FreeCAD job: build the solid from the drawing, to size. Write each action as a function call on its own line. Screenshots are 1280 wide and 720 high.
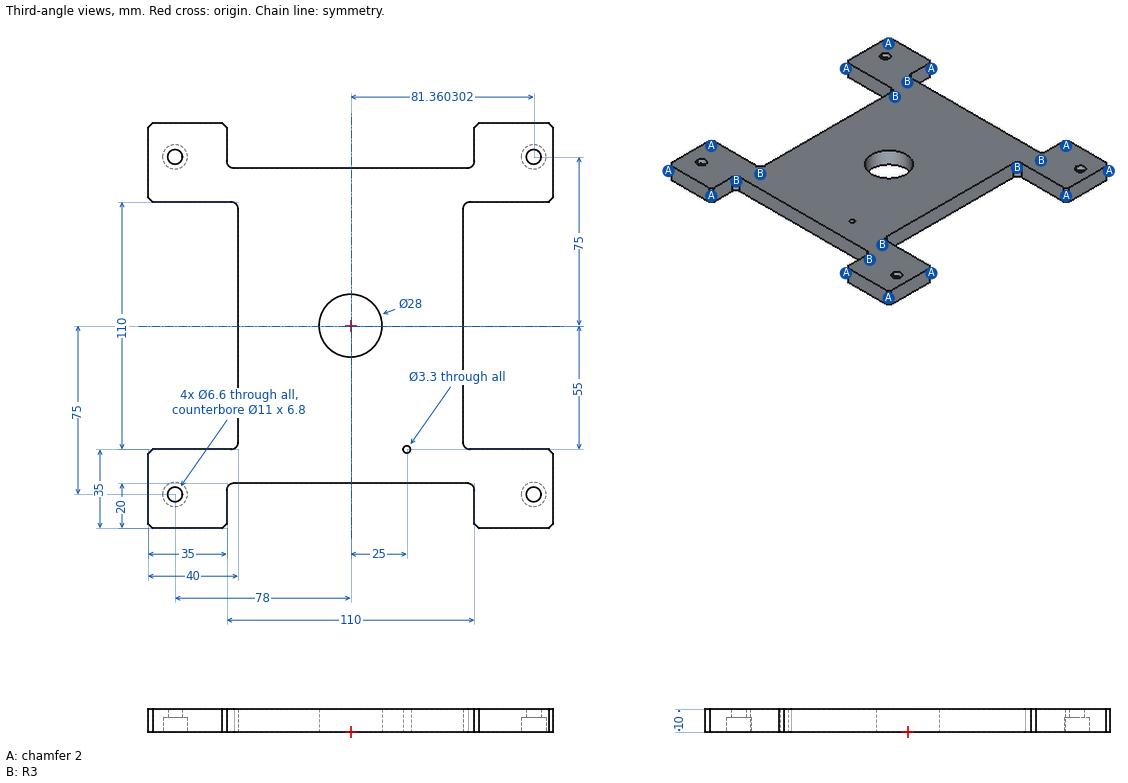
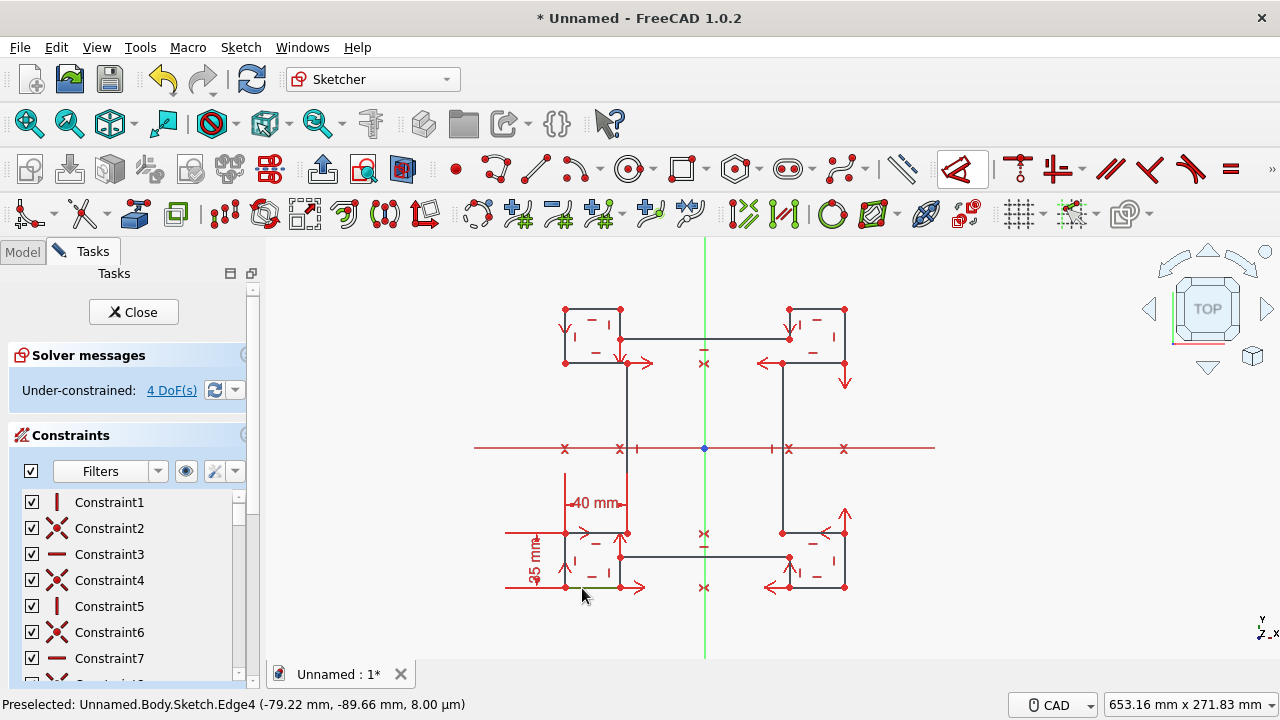
click(982, 170)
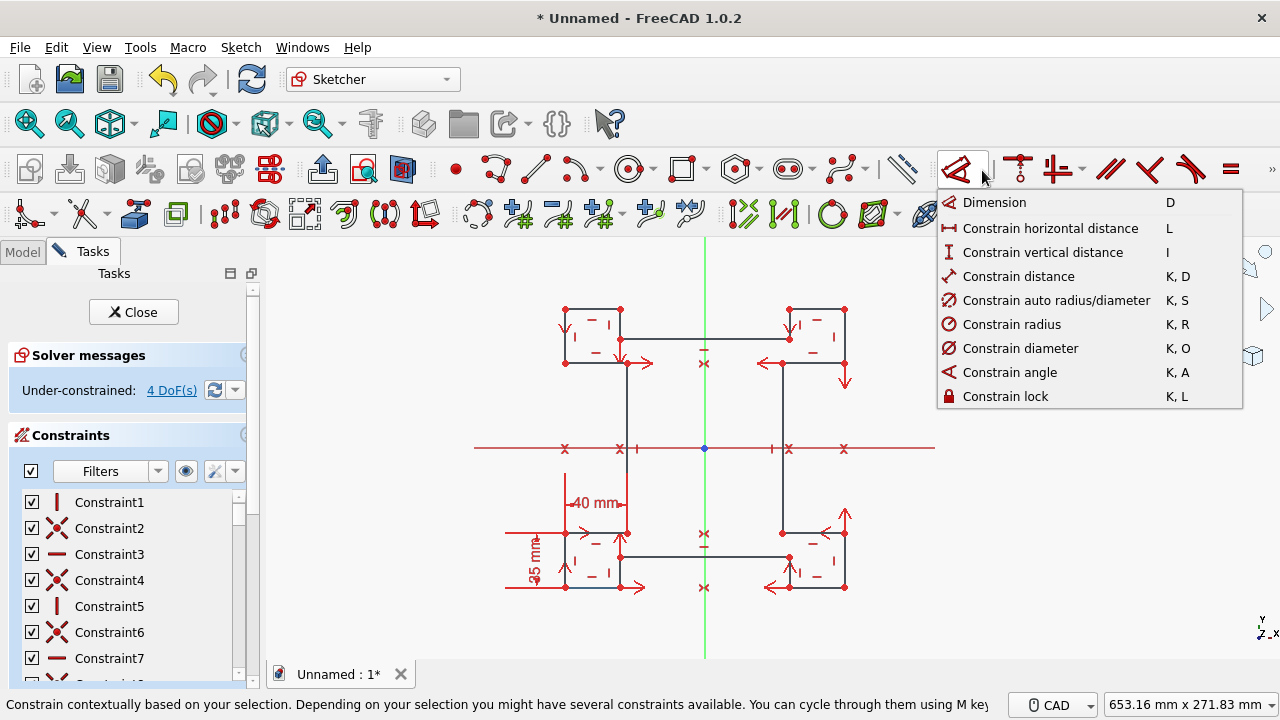
click(1090, 228)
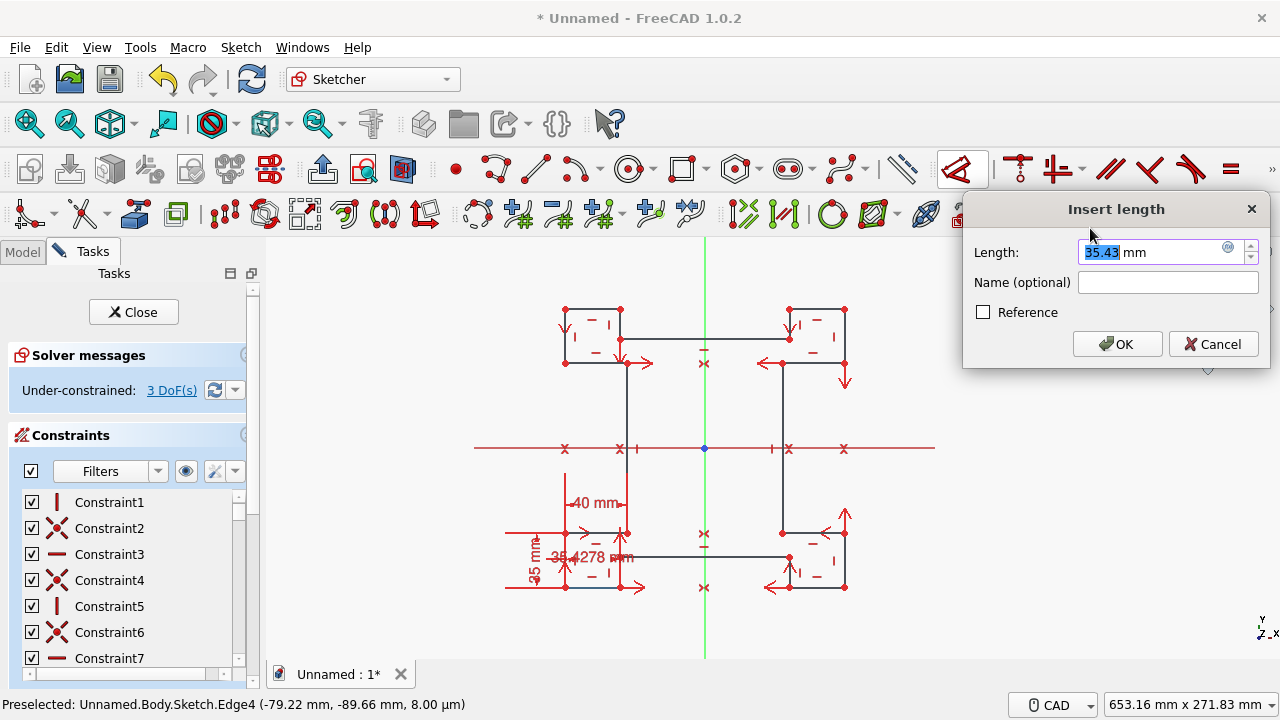
text(35)
key(Return)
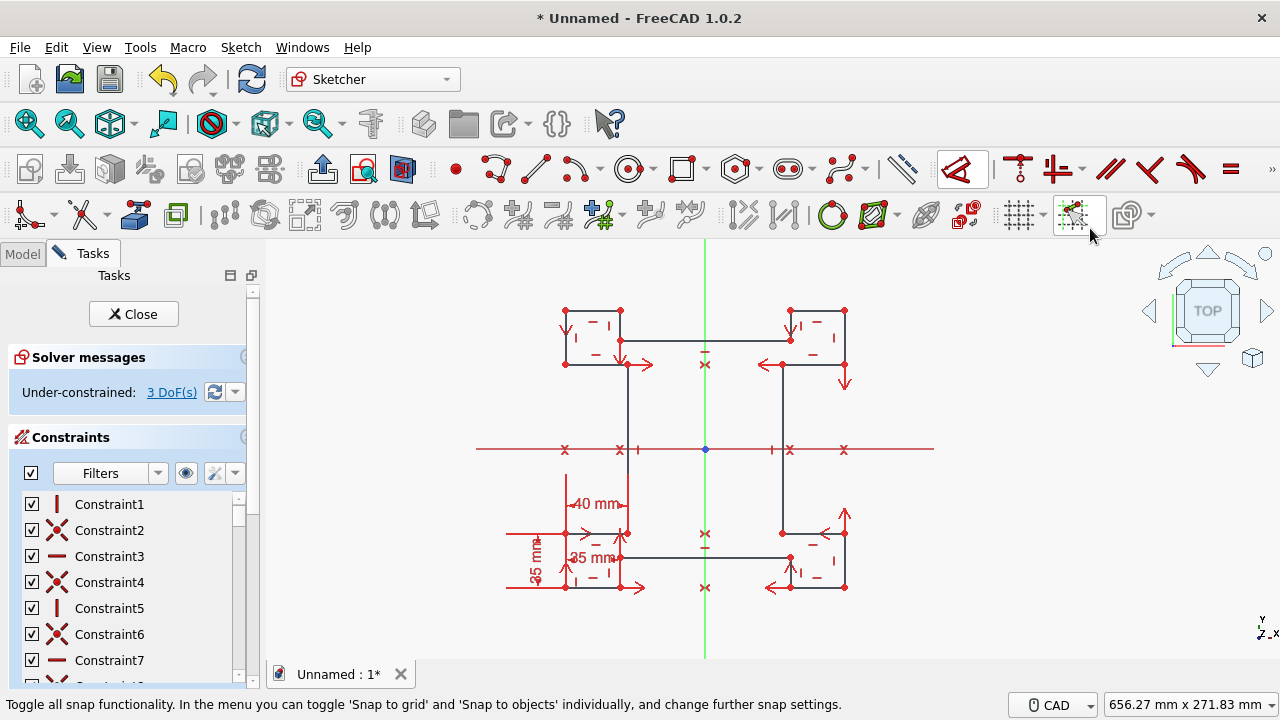
scroll(620, 576, up, 2)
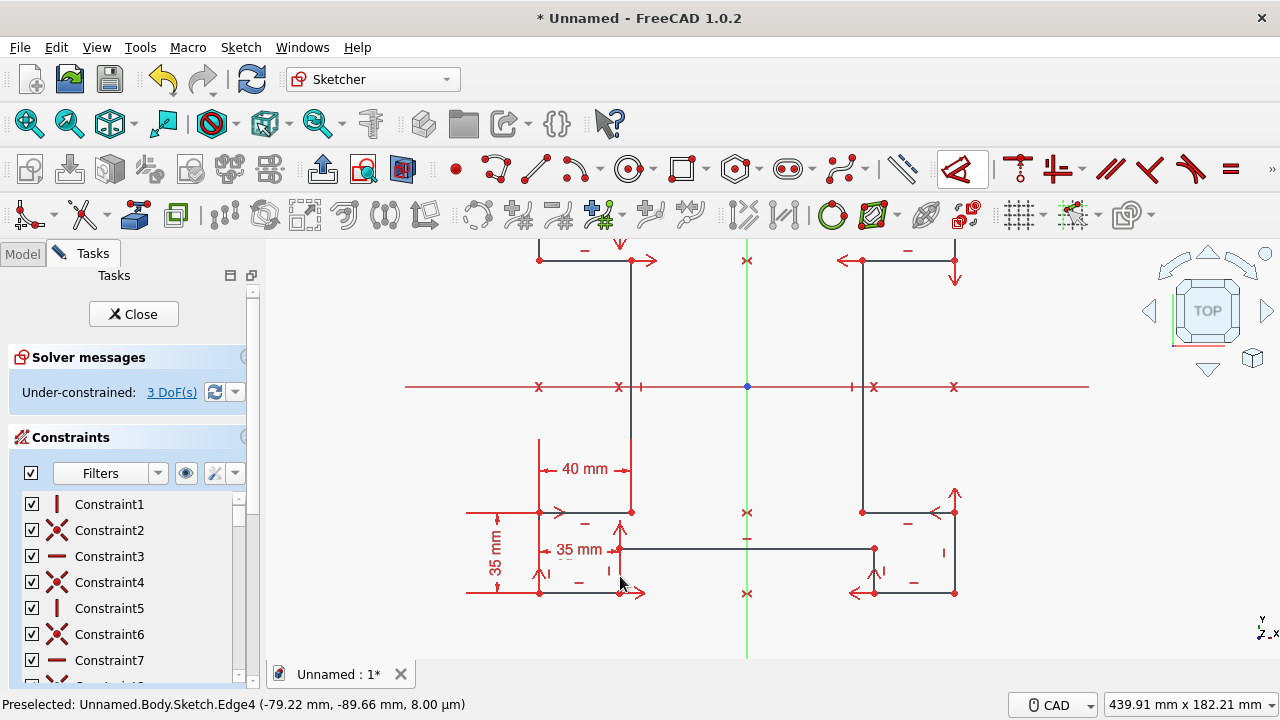
click(620, 575)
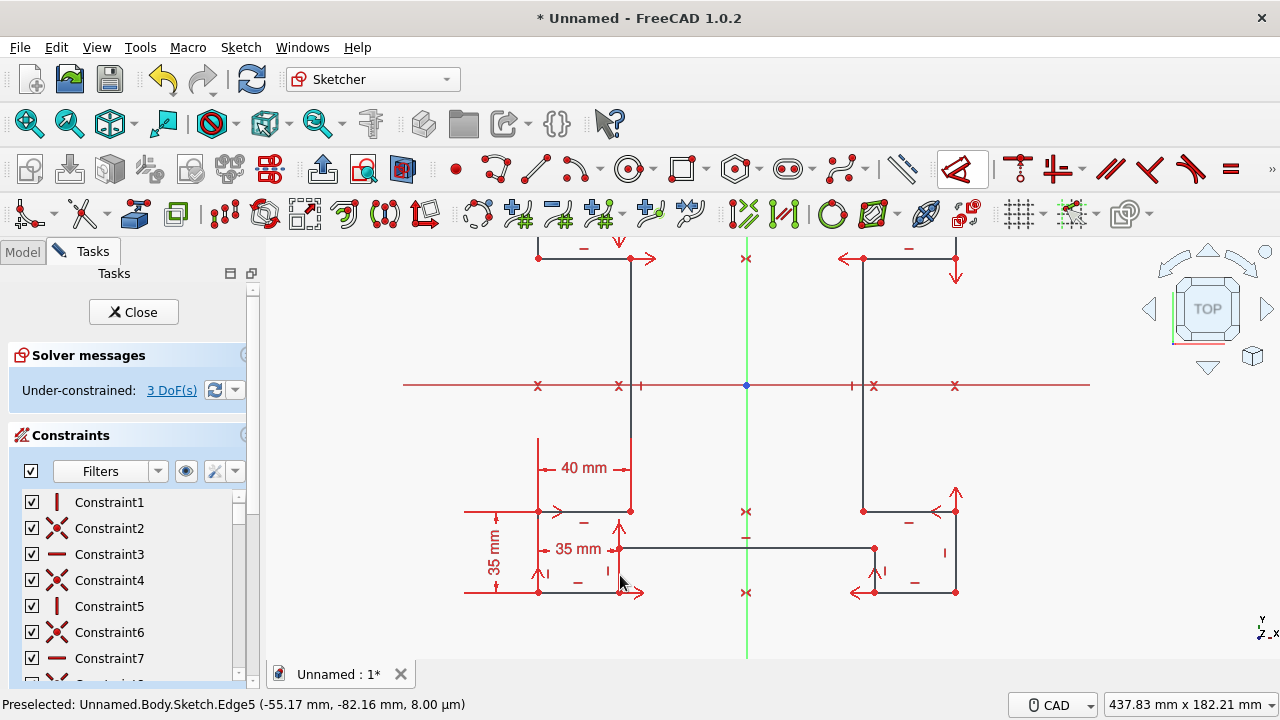
click(982, 170)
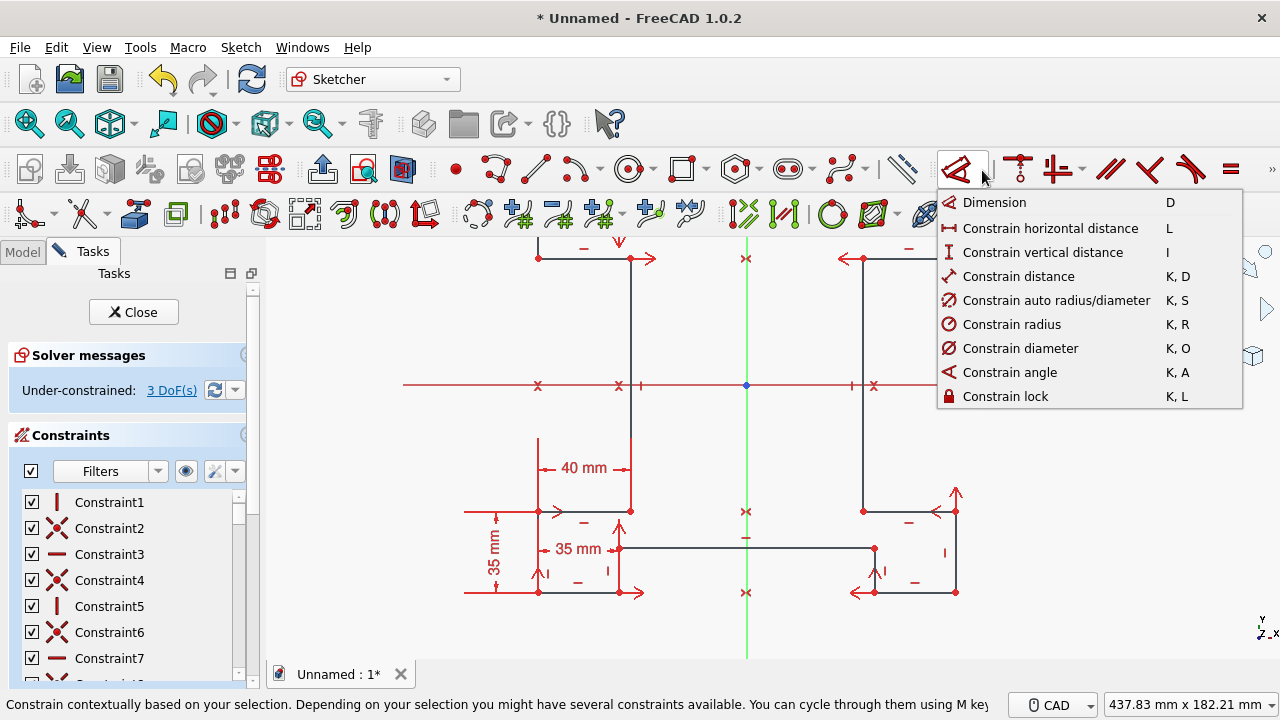
click(1090, 252)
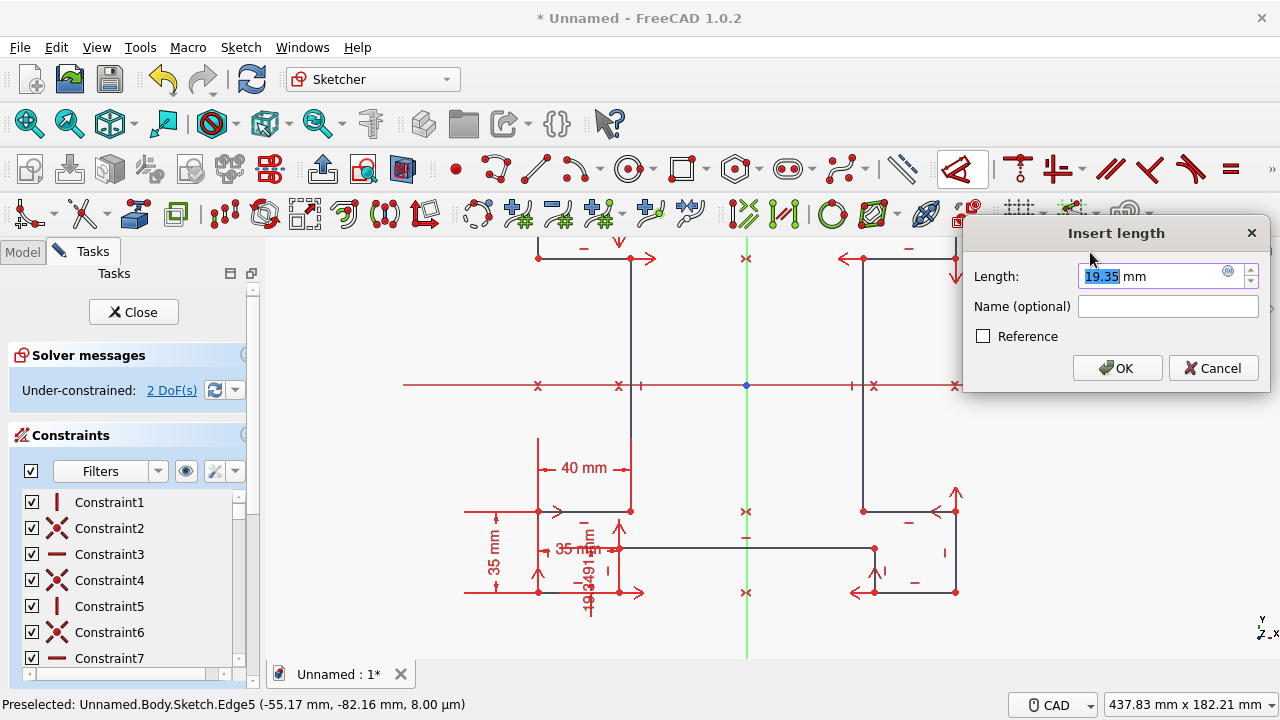
text(20)
key(Return)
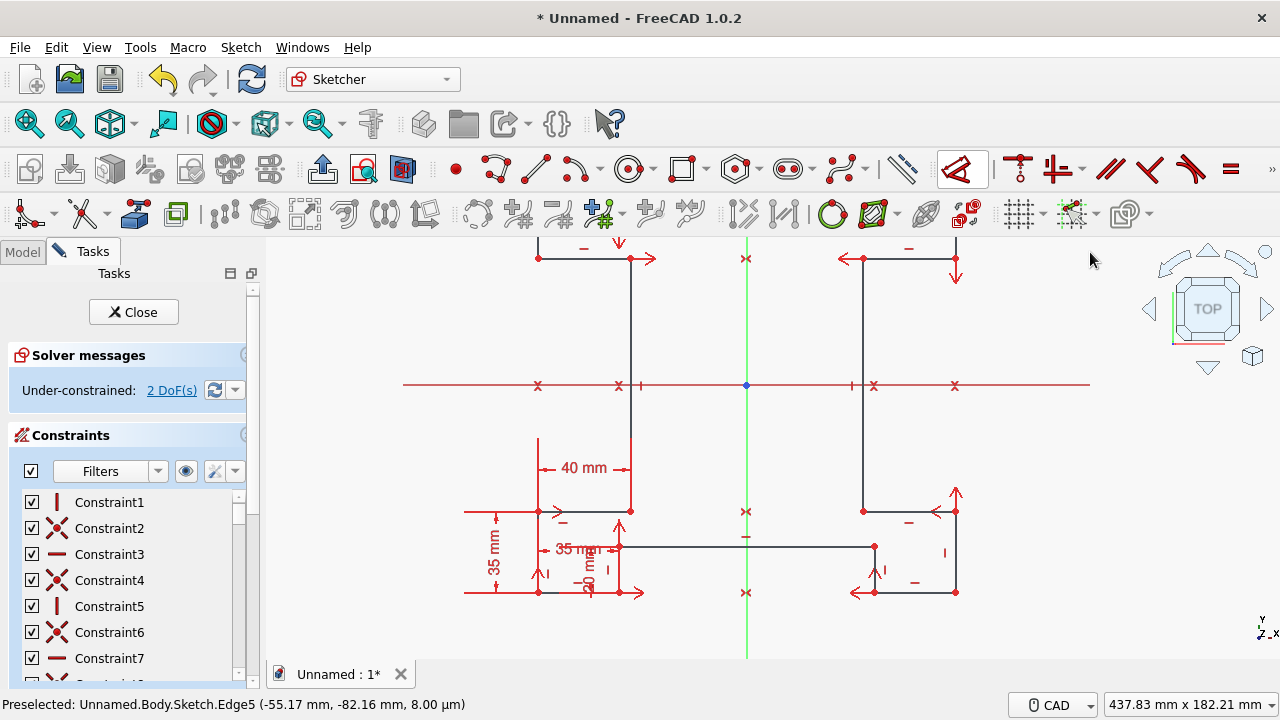
click(631, 335)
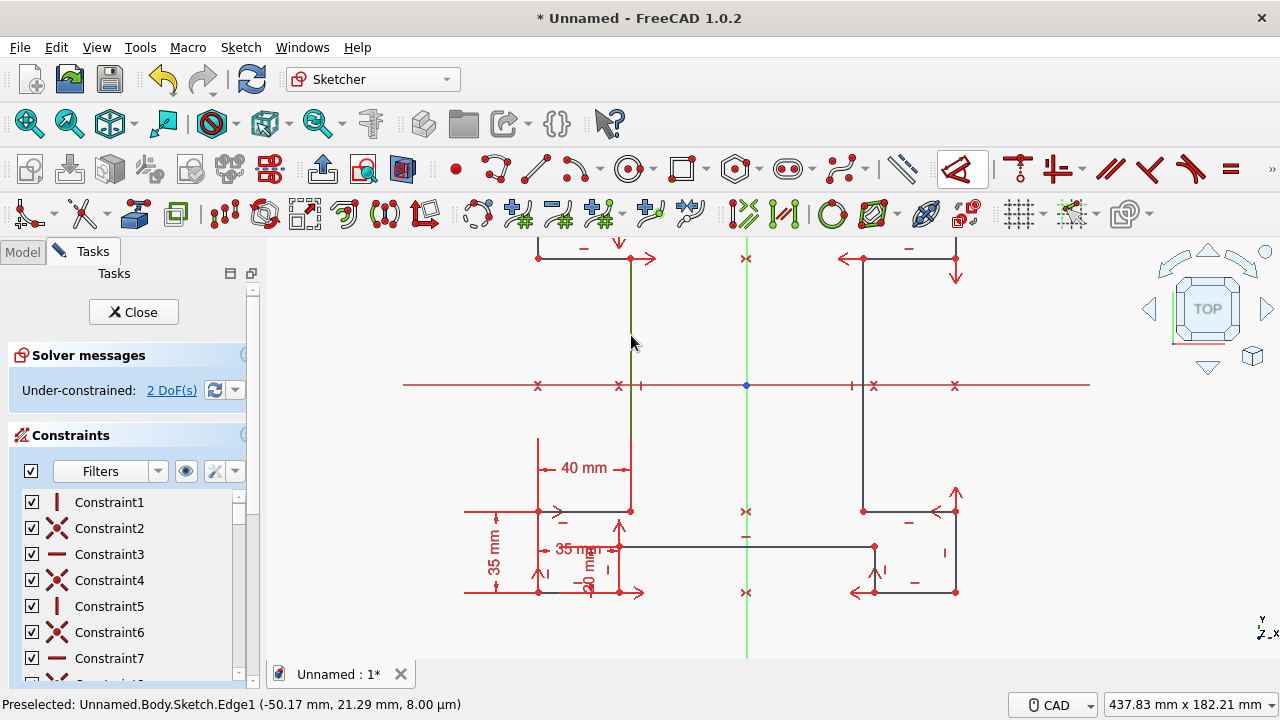
click(982, 170)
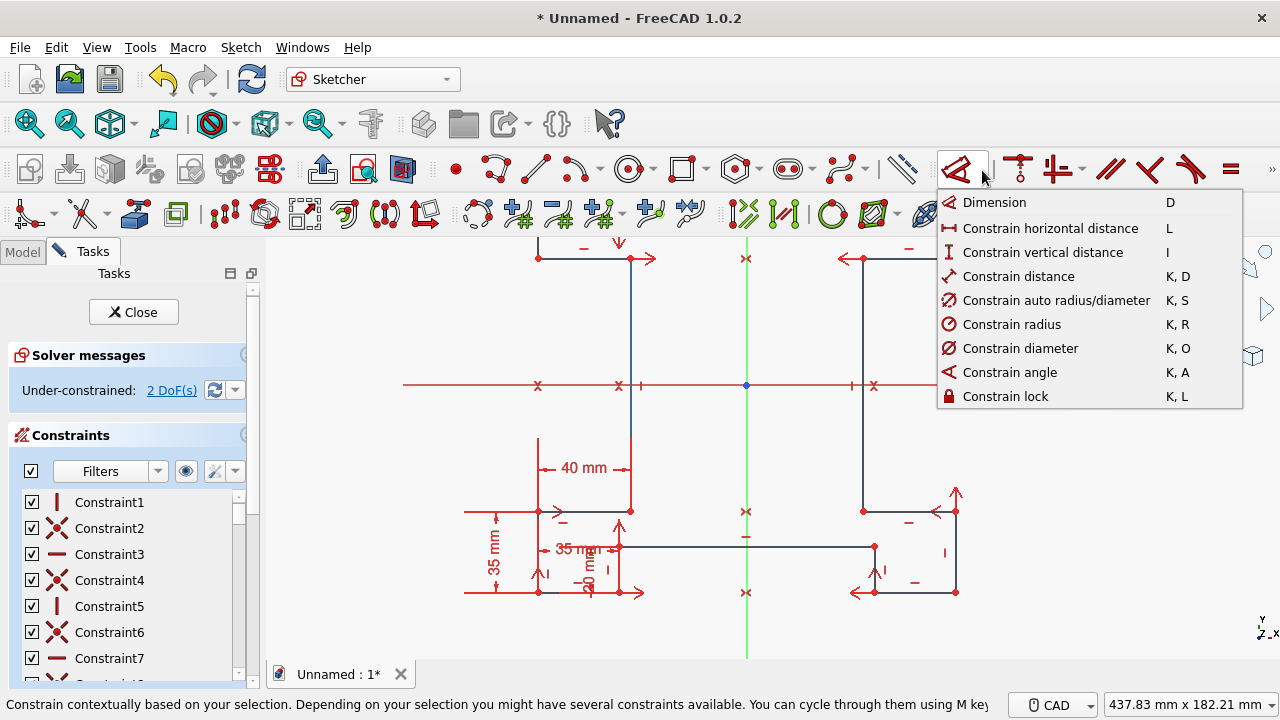
click(1090, 252)